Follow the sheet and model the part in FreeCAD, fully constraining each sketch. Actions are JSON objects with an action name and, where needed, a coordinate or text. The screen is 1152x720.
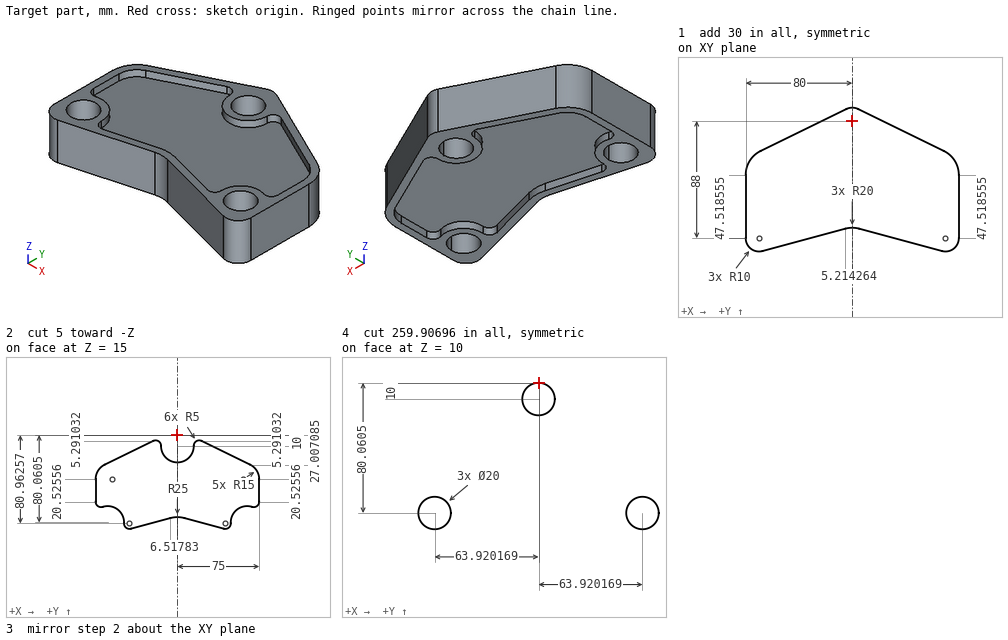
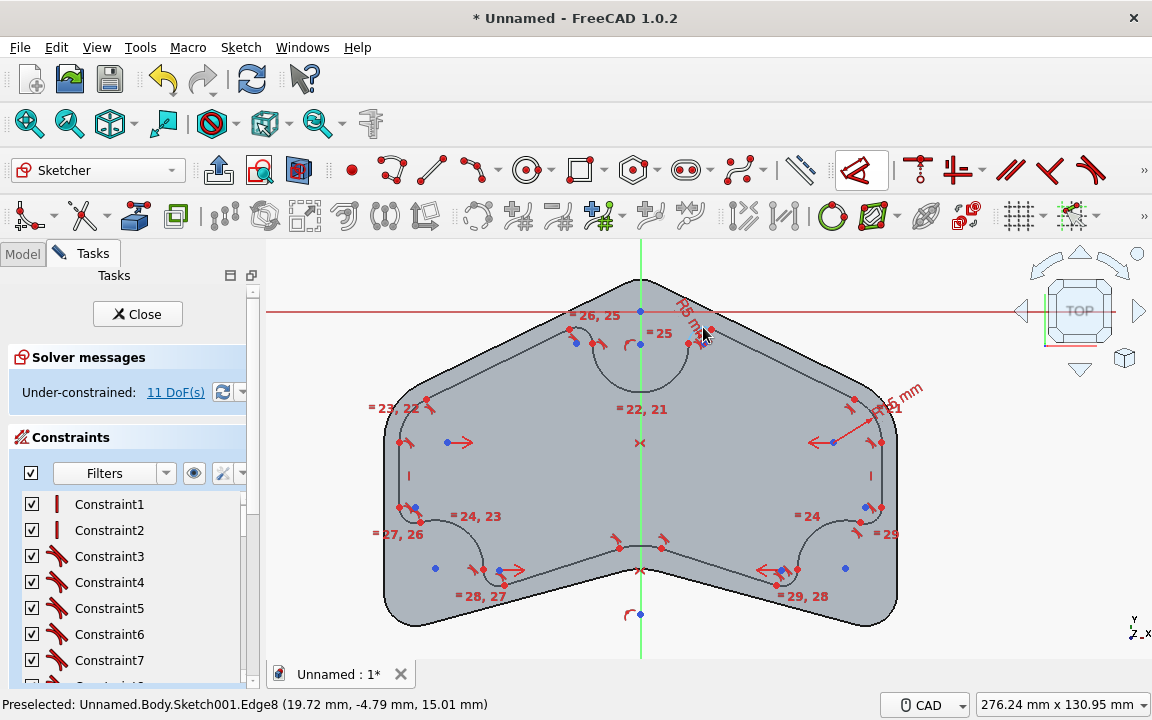
{"action": "scroll", "coordinate": [649, 546], "scroll_direction": "up", "scroll_amount": 3}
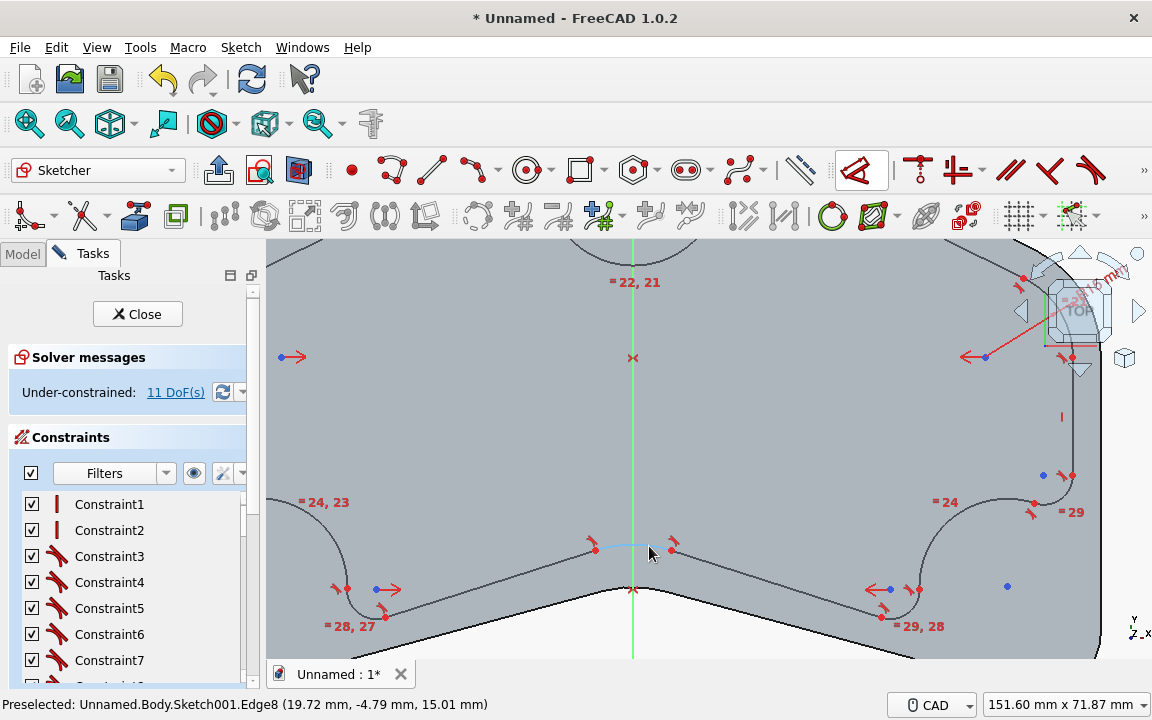
{"action": "left_click", "coordinate": [649, 546]}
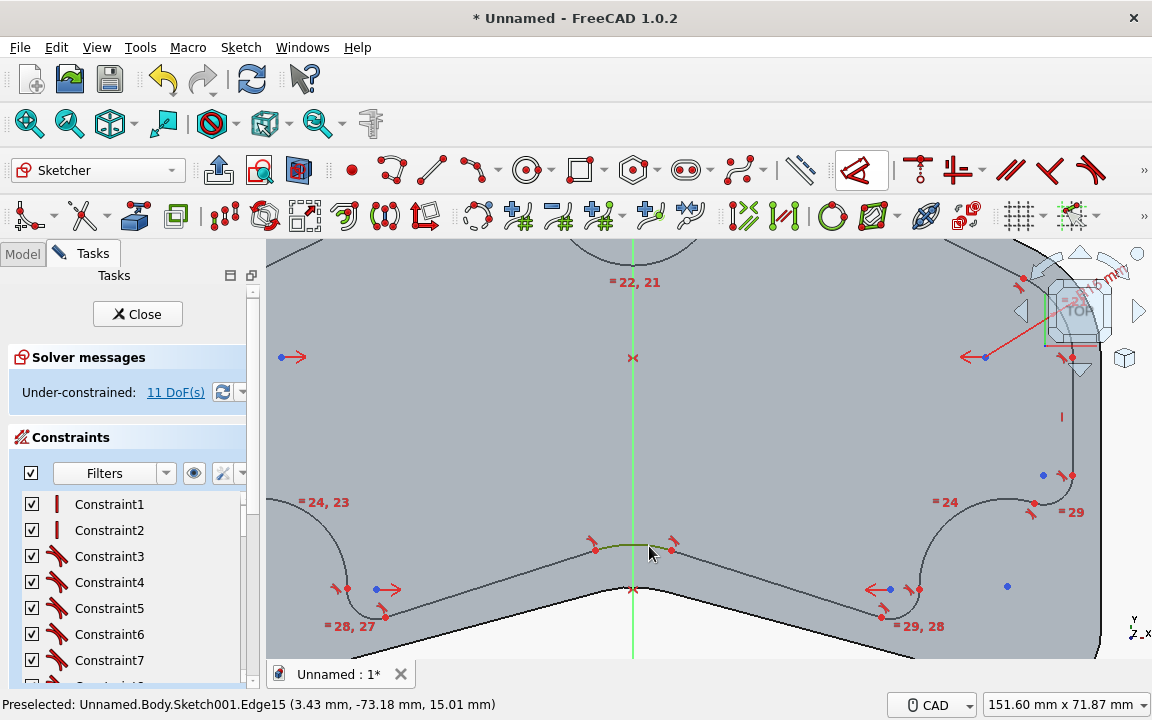
{"action": "left_click", "coordinate": [882, 170]}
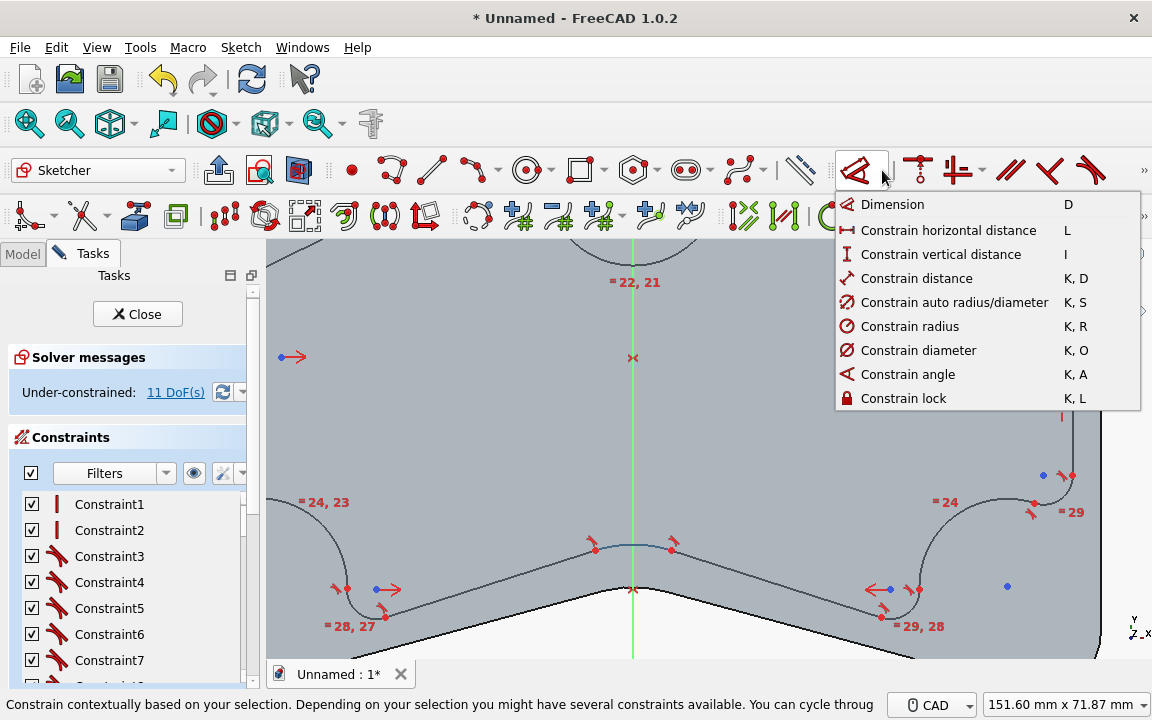
{"action": "left_click", "coordinate": [988, 326]}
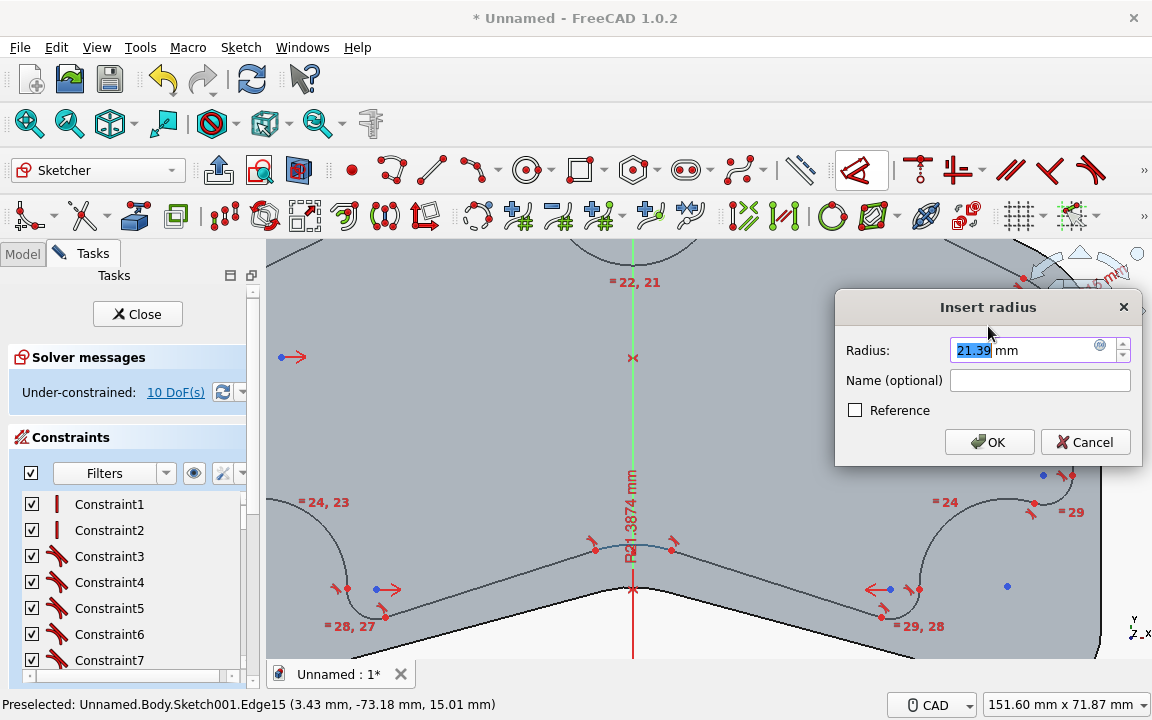
{"action": "type", "text": "25"}
{"action": "key", "text": "Return"}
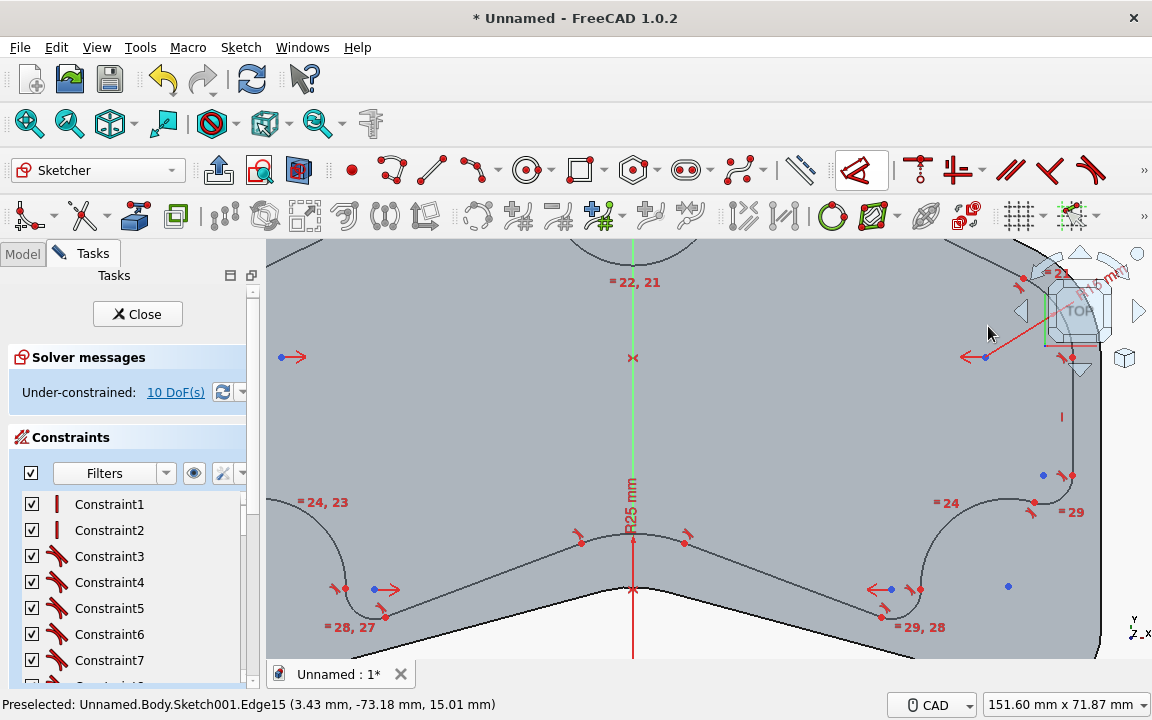
{"action": "scroll", "coordinate": [649, 546], "scroll_direction": "down", "scroll_amount": 3}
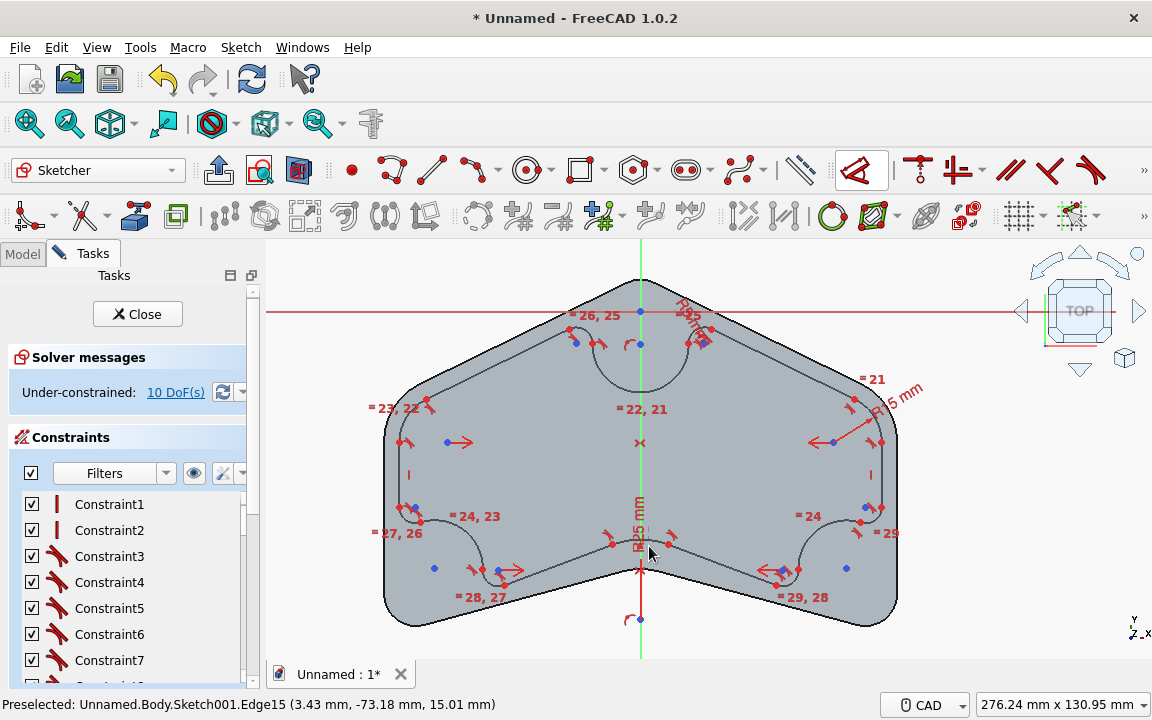
{"action": "left_click", "coordinate": [882, 507]}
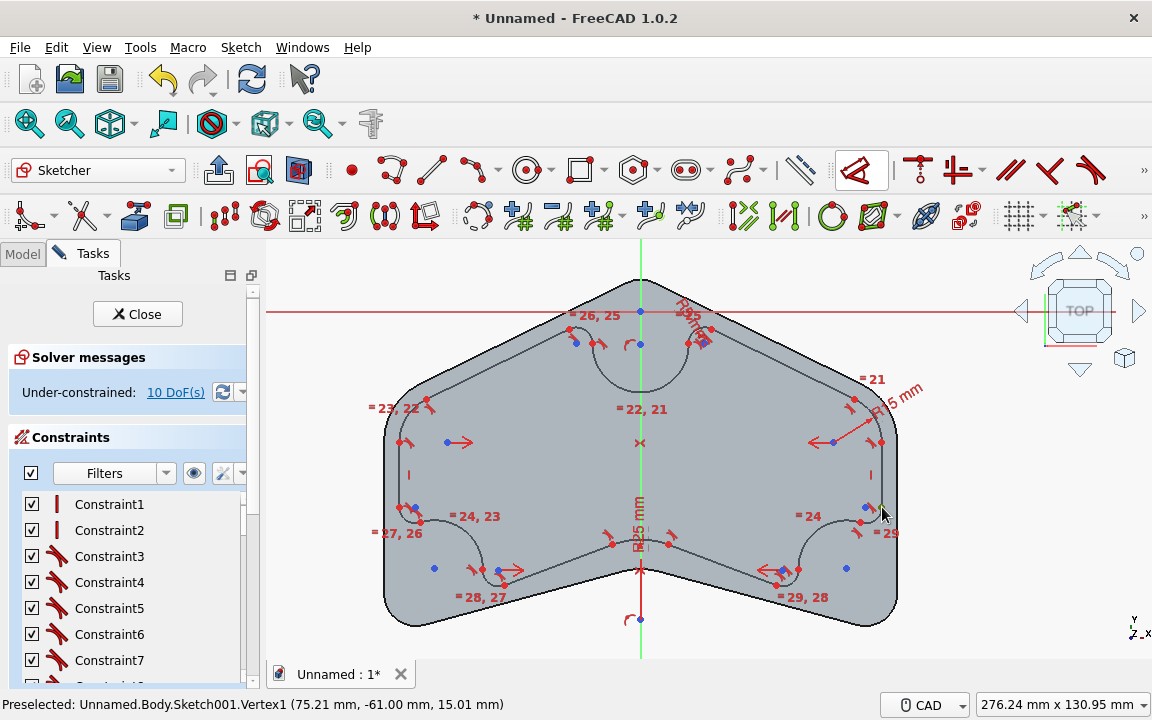
{"action": "left_click", "coordinate": [882, 170]}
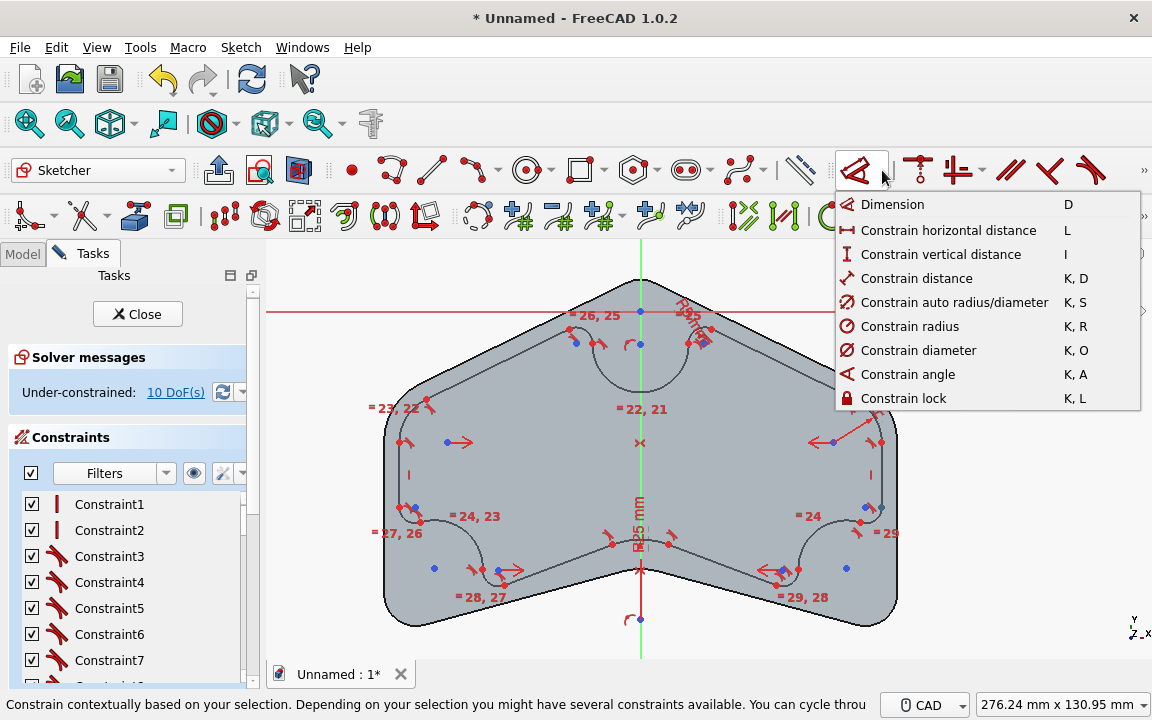
{"action": "left_click", "coordinate": [988, 230]}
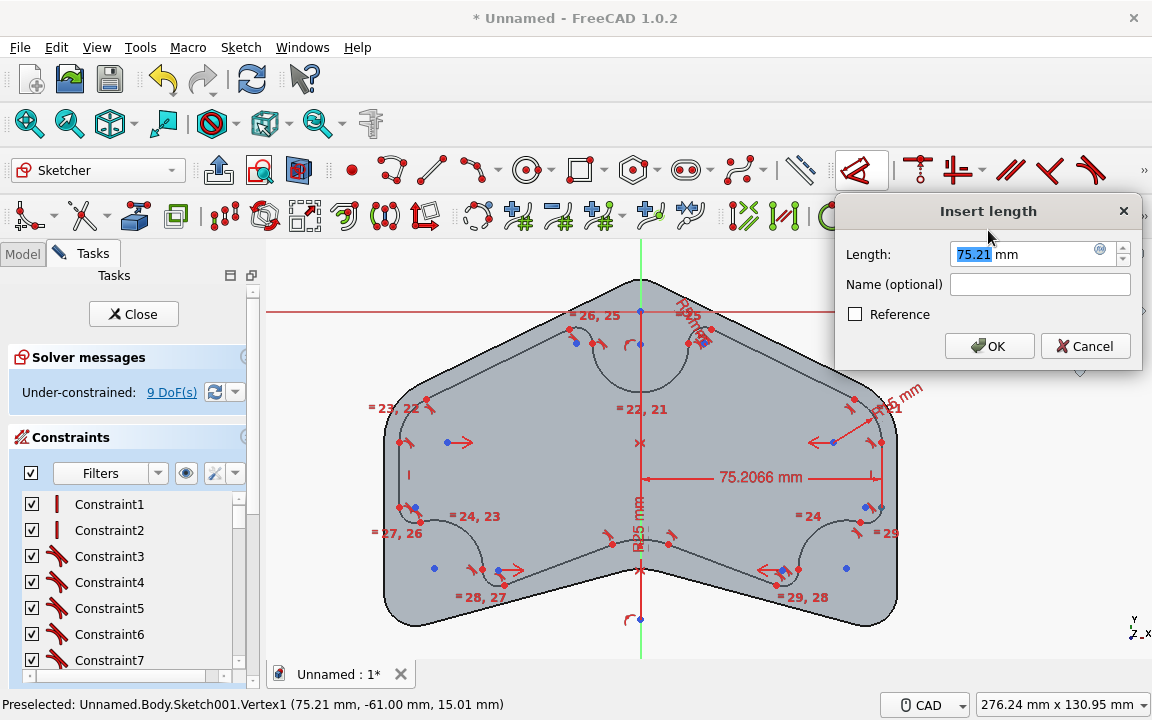
{"action": "type", "text": "75"}
{"action": "key", "text": "Return"}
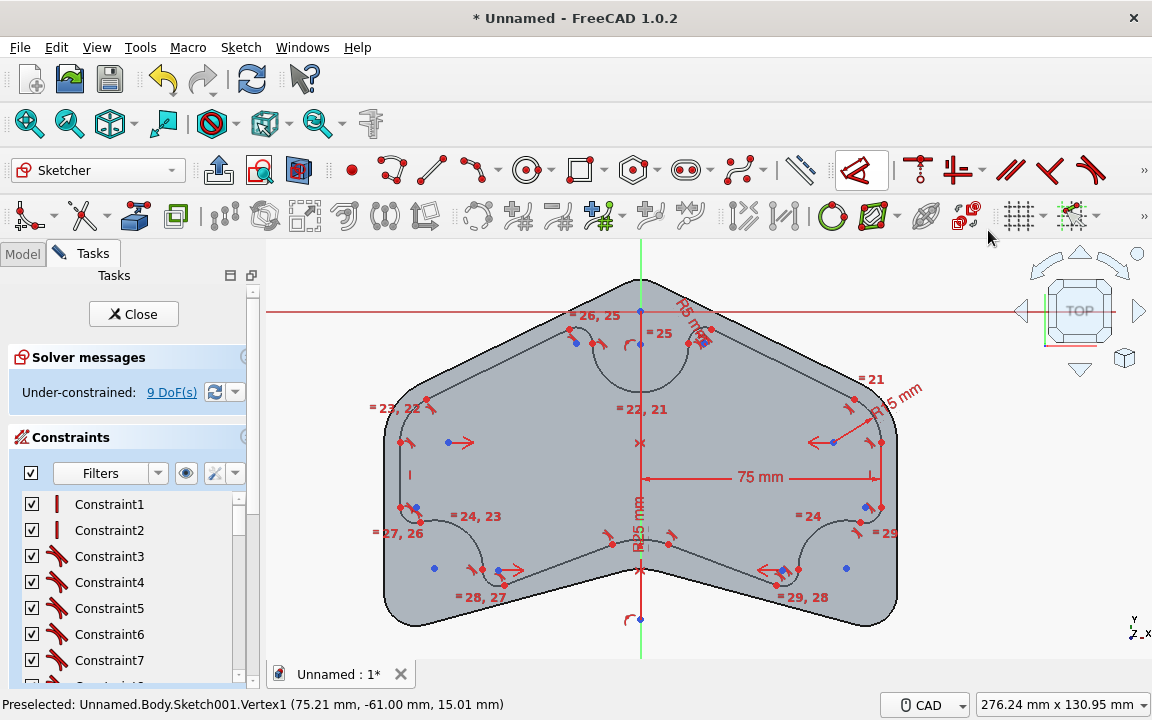
{"action": "scroll", "coordinate": [641, 344], "scroll_direction": "up", "scroll_amount": 2}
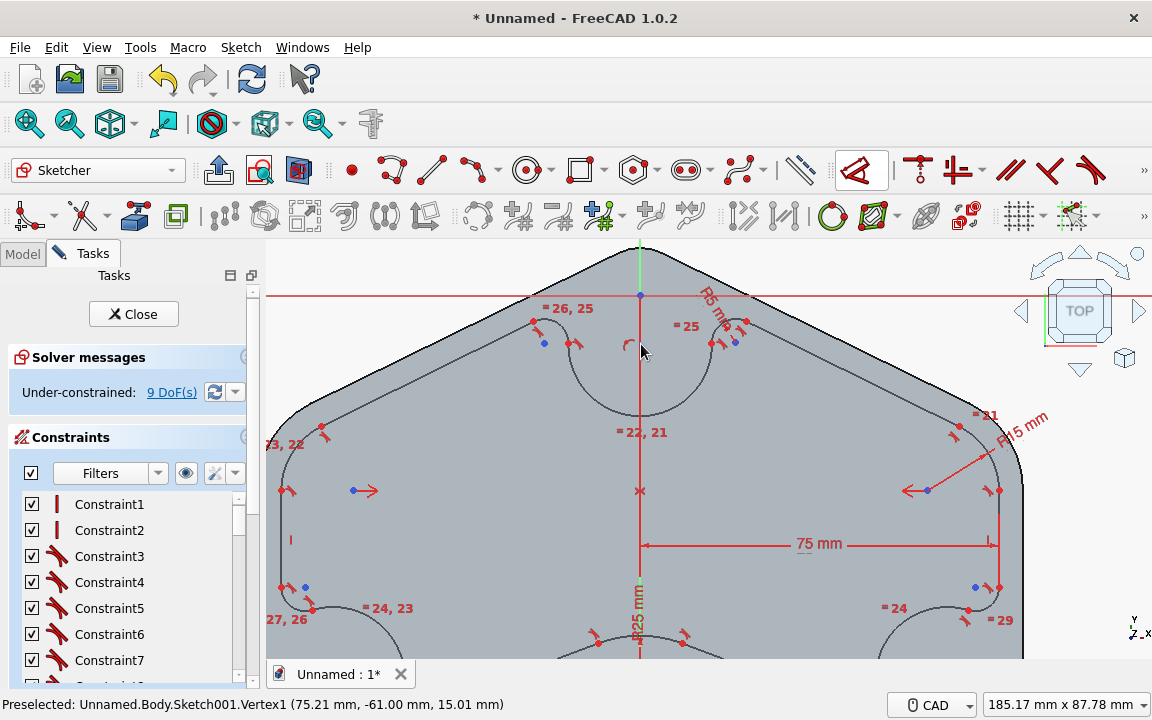
{"action": "left_click", "coordinate": [640, 344]}